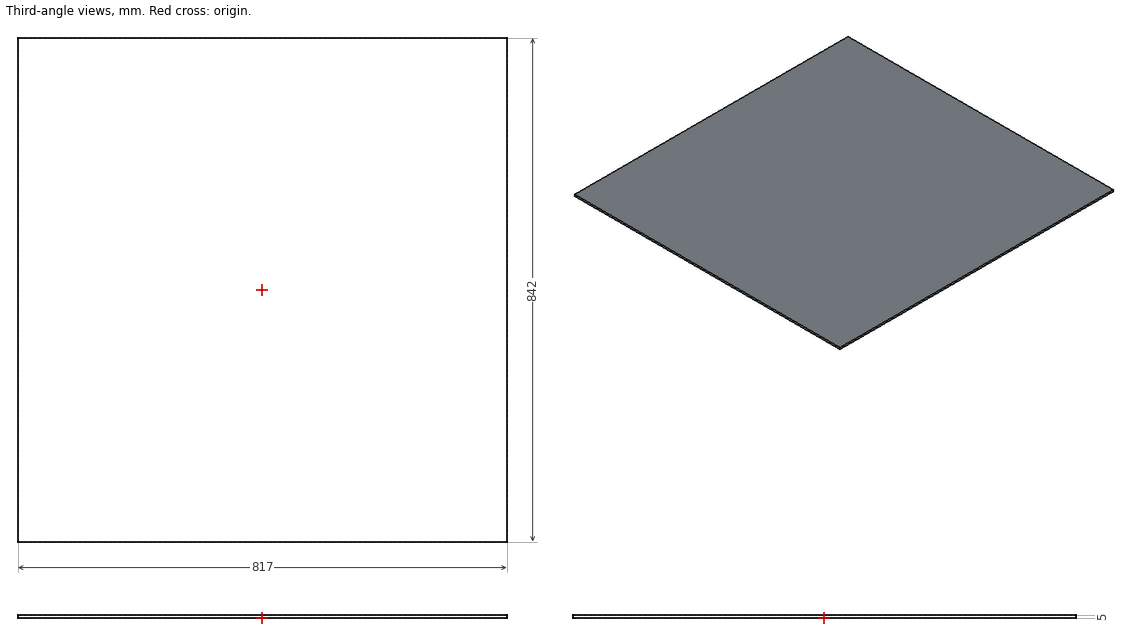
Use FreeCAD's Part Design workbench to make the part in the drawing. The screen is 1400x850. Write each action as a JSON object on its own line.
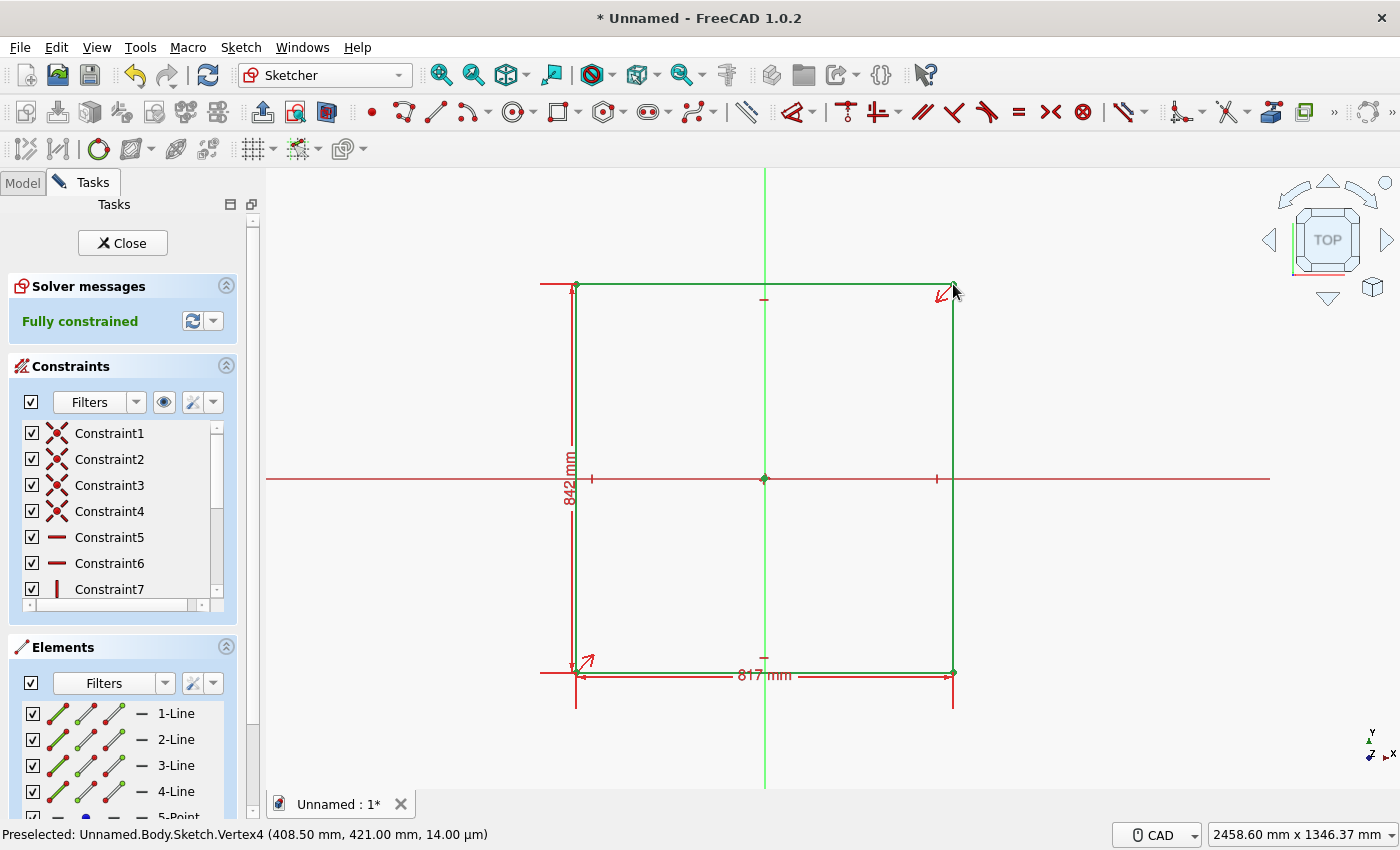
{"action": "left_click", "coordinate": [123, 243]}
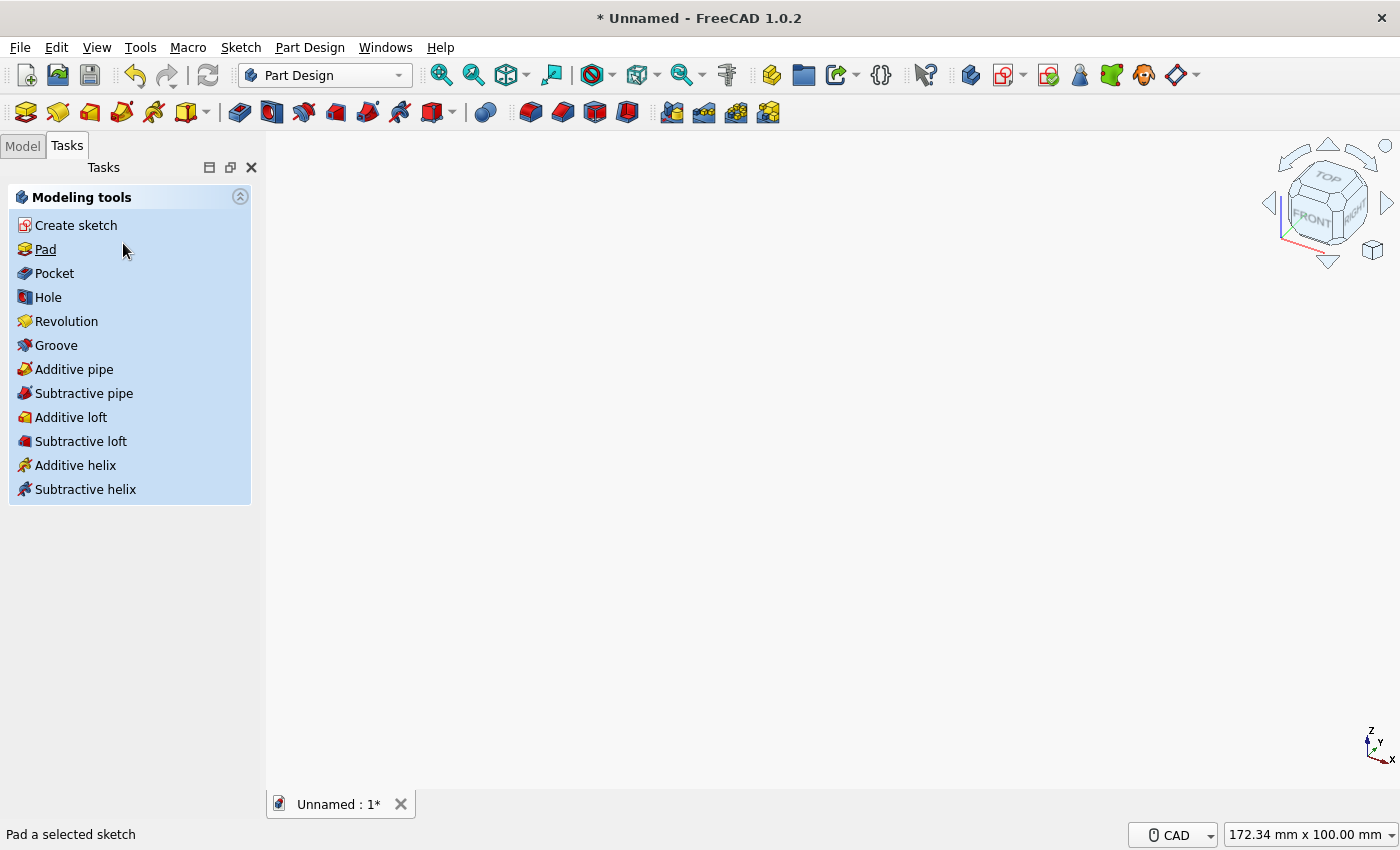
{"action": "left_click", "coordinate": [26, 112]}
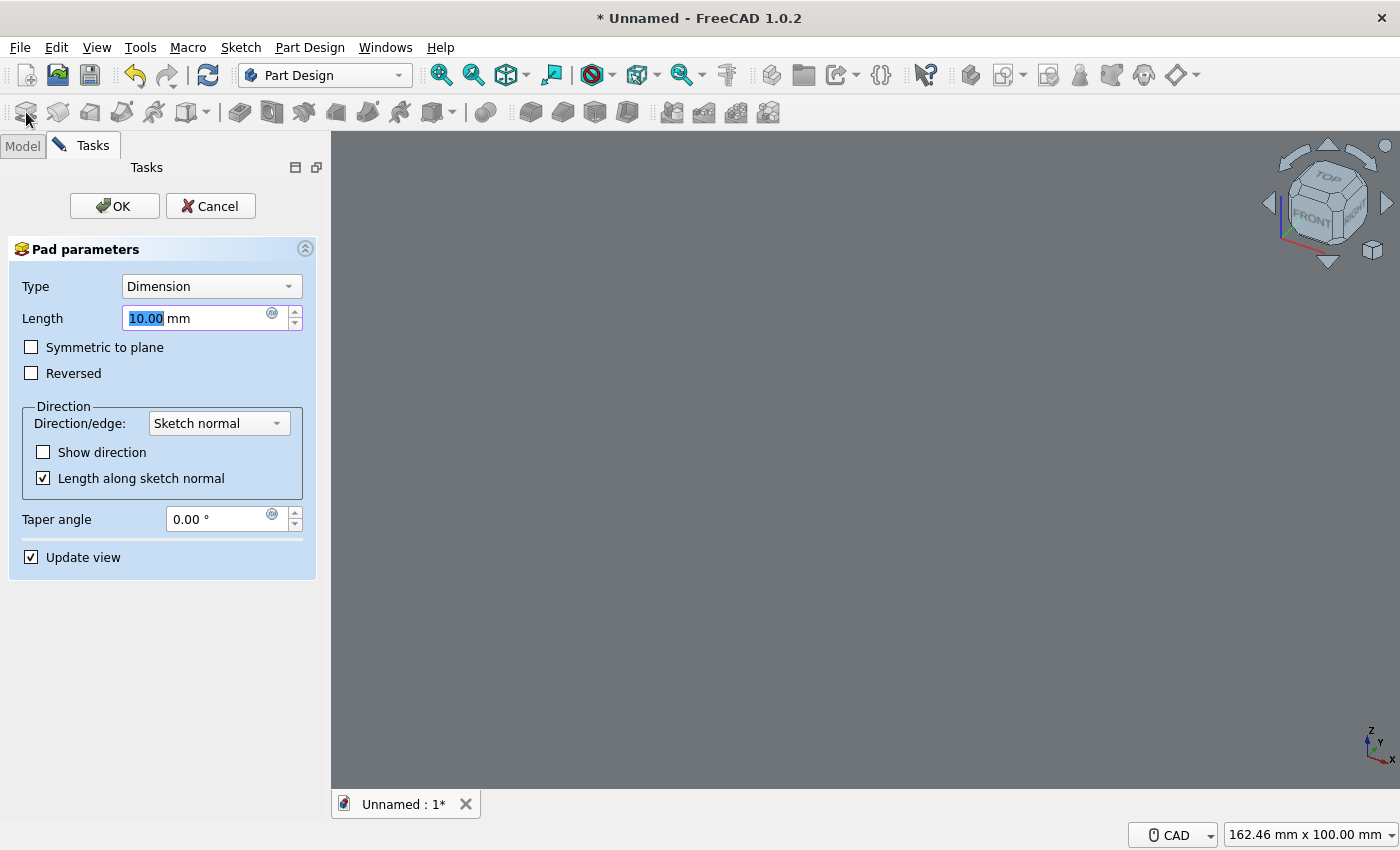
{"action": "type", "text": "5"}
{"action": "key", "text": "Tab"}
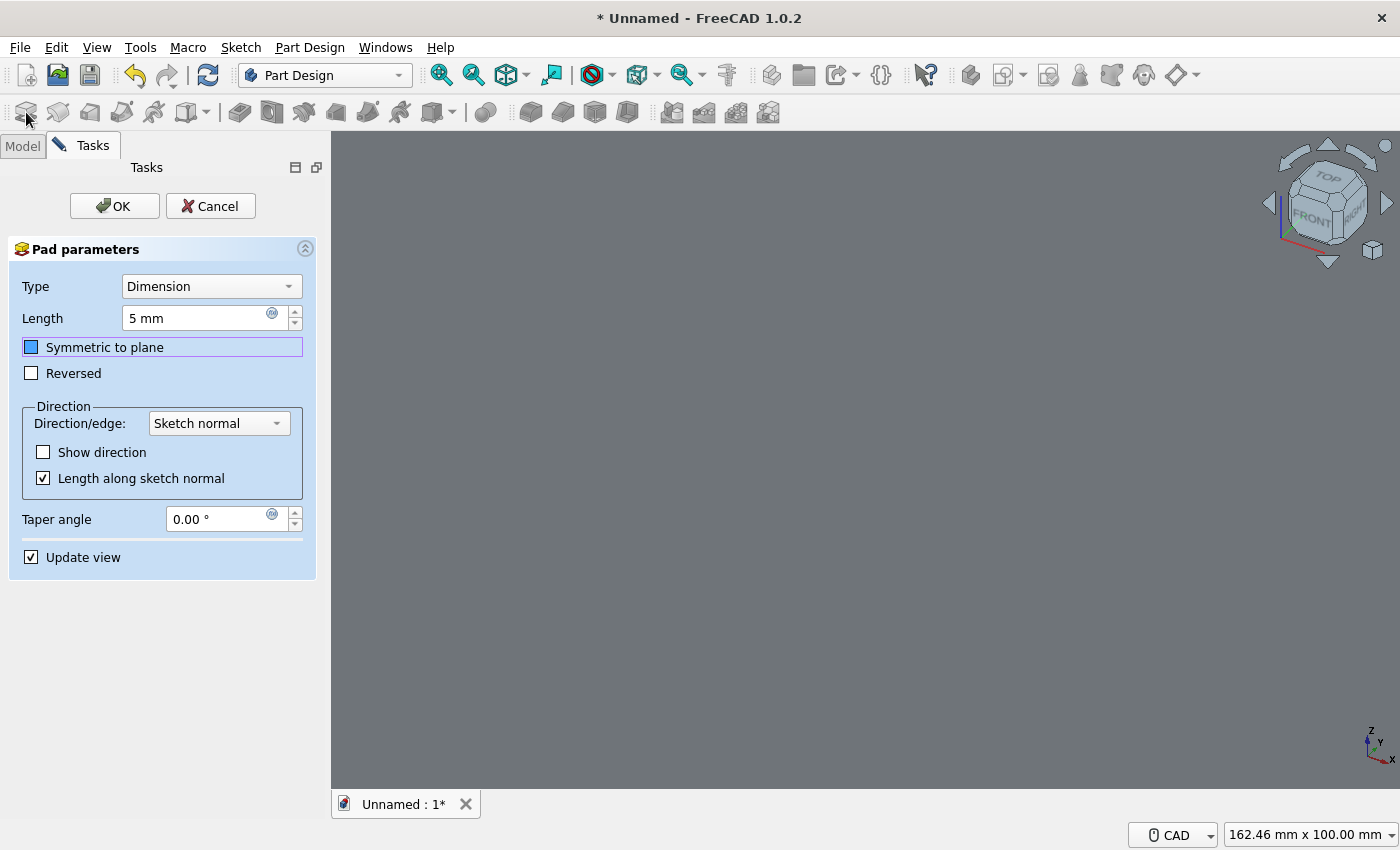
{"action": "left_click", "coordinate": [115, 206]}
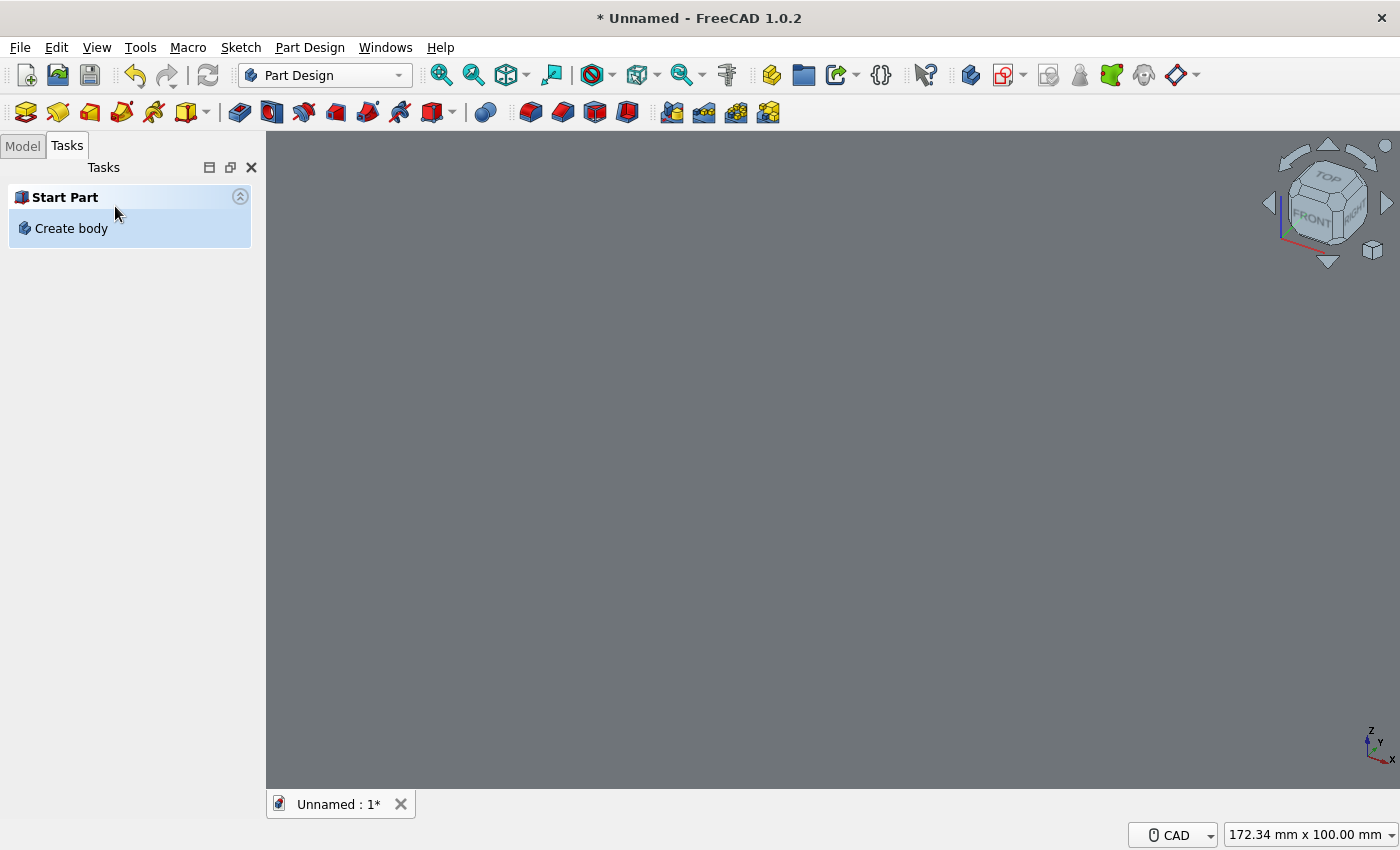
{"action": "key", "text": "0"}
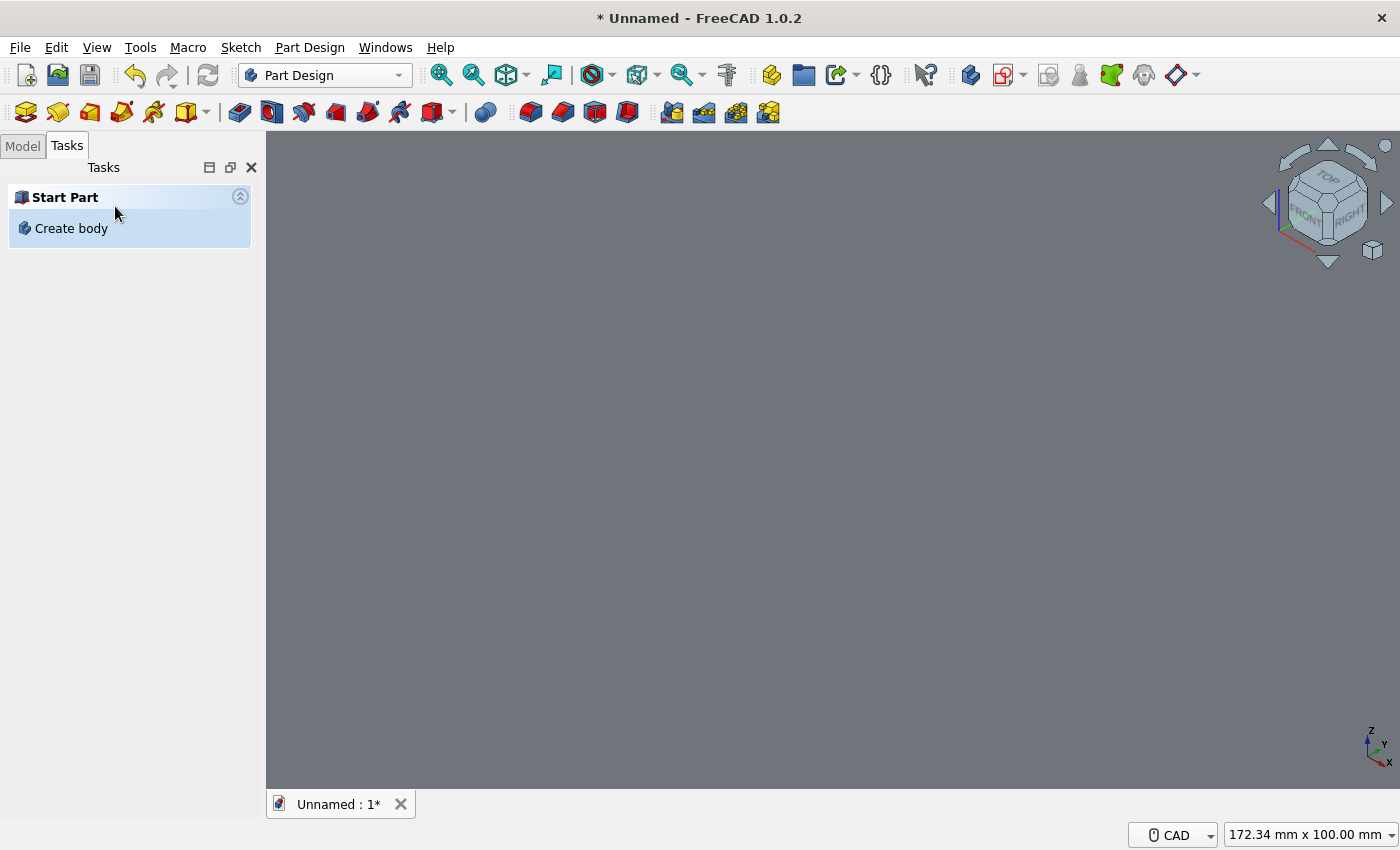
{"action": "key", "text": "v f"}